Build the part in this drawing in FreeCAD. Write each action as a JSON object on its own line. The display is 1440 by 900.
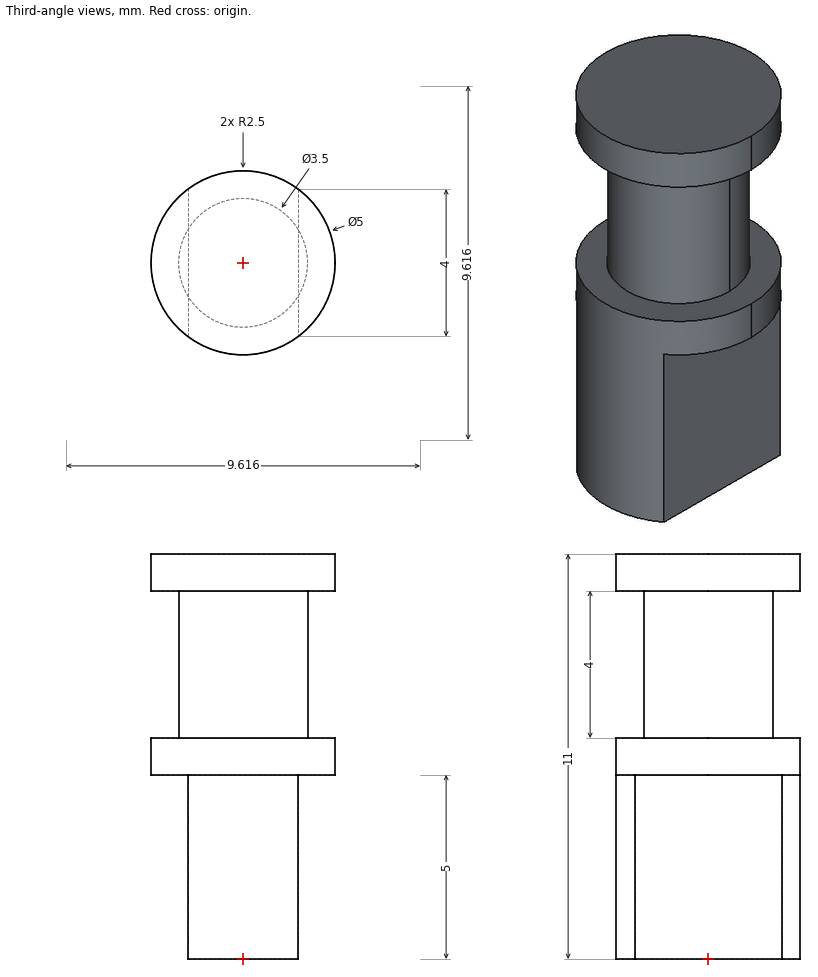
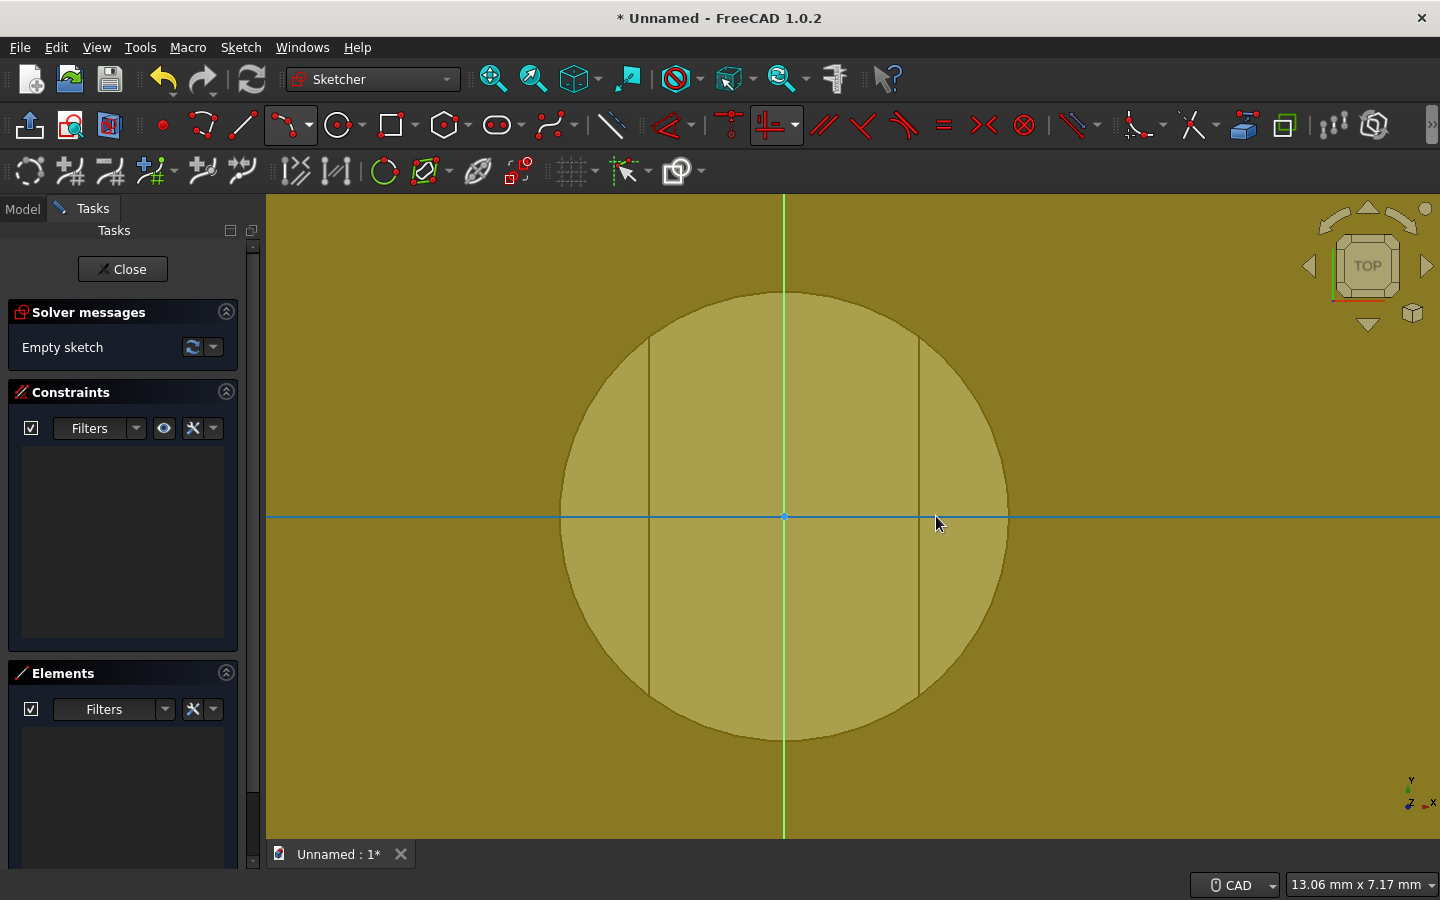
{"action": "key", "text": "g c"}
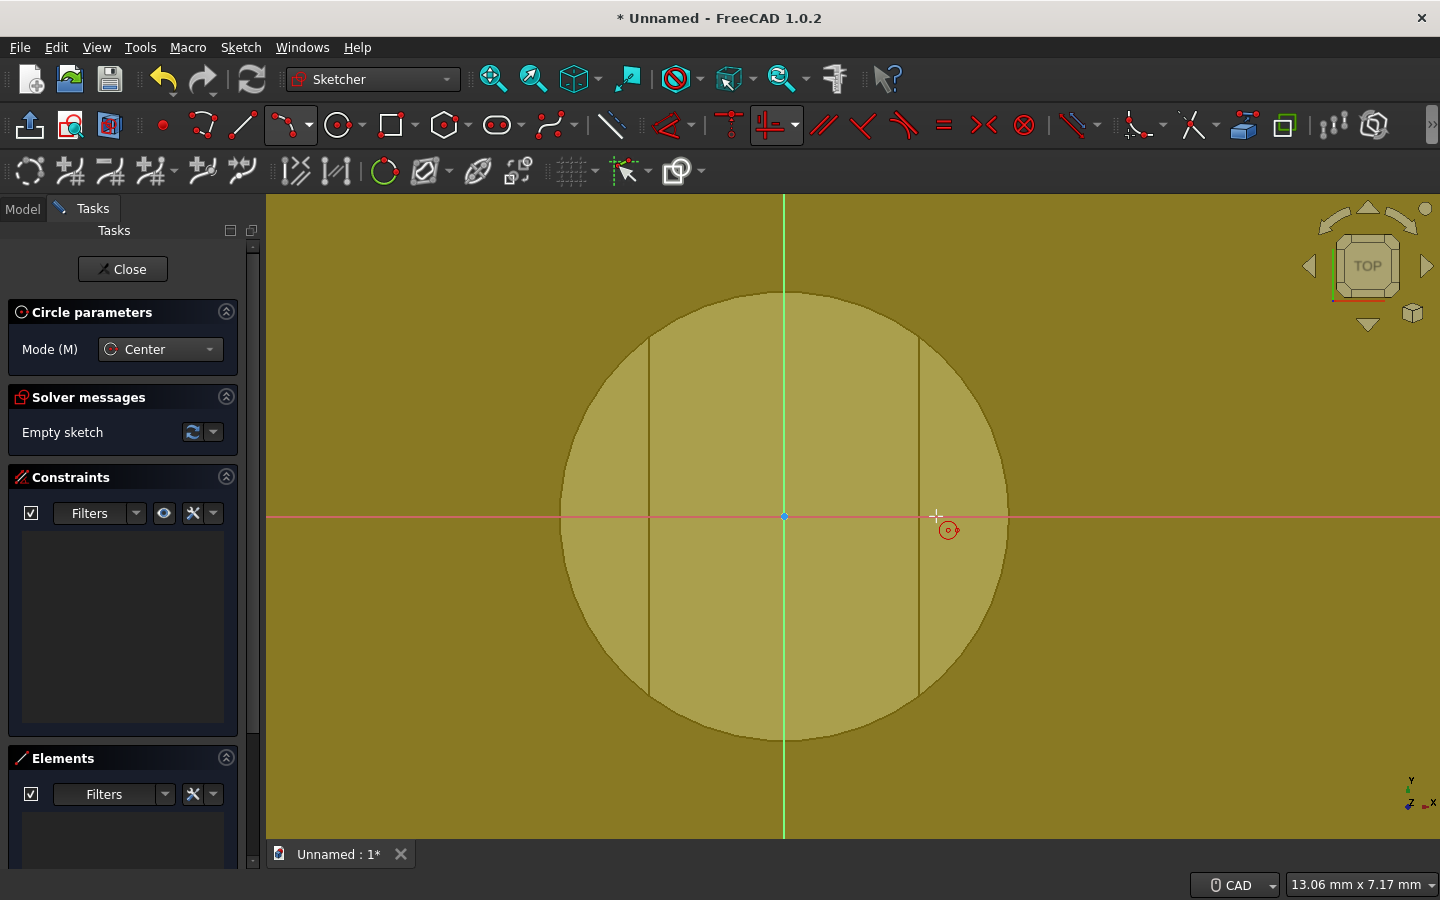
{"action": "left_click", "coordinate": [784, 516]}
{"action": "mouse_move", "coordinate": [943, 358]}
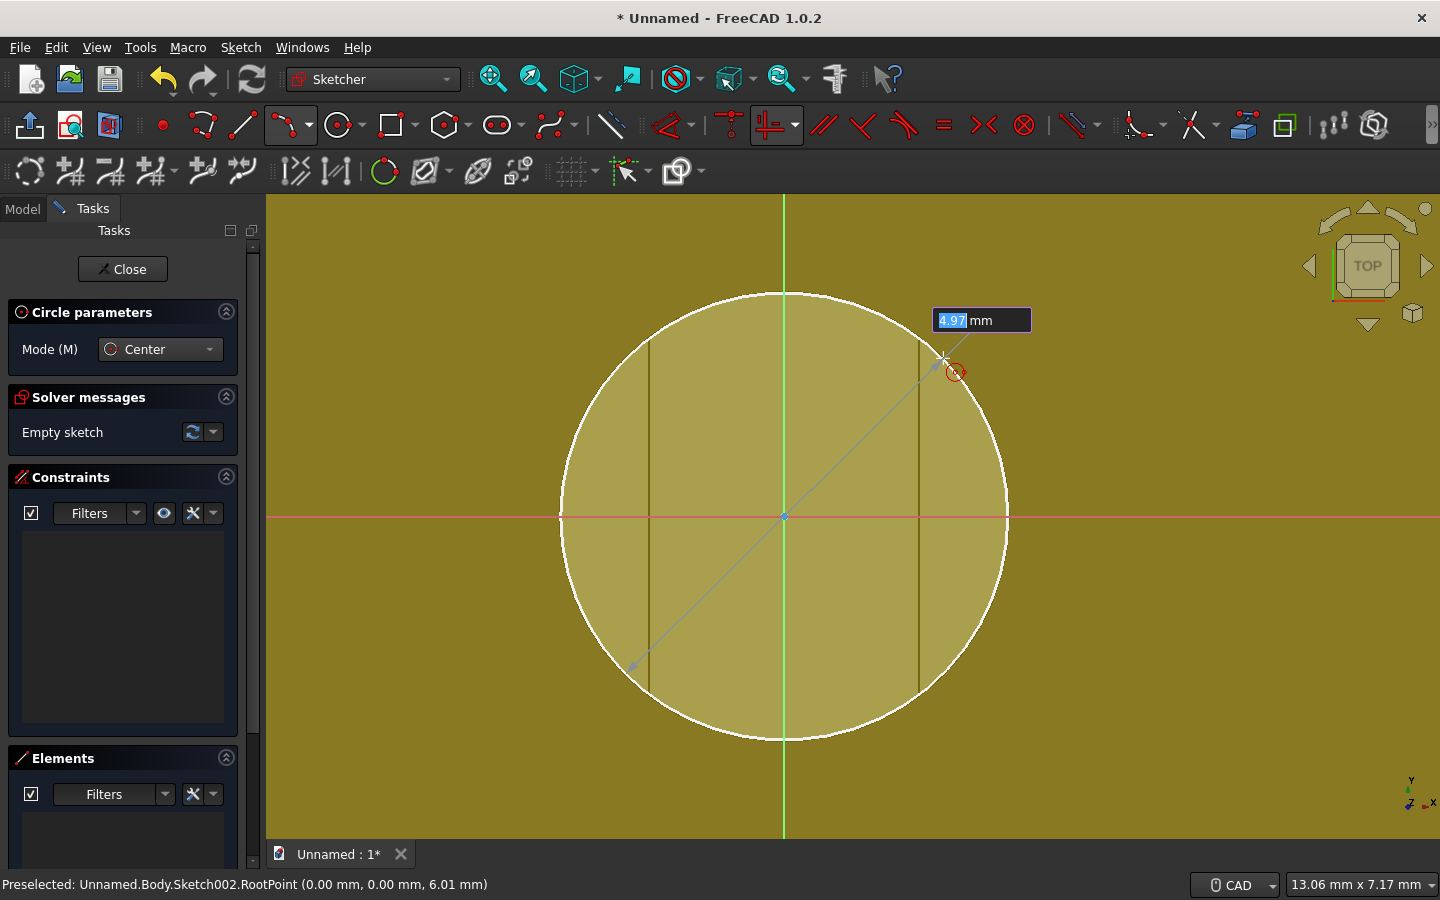
{"action": "type", "text": "5"}
{"action": "key", "text": "Return"}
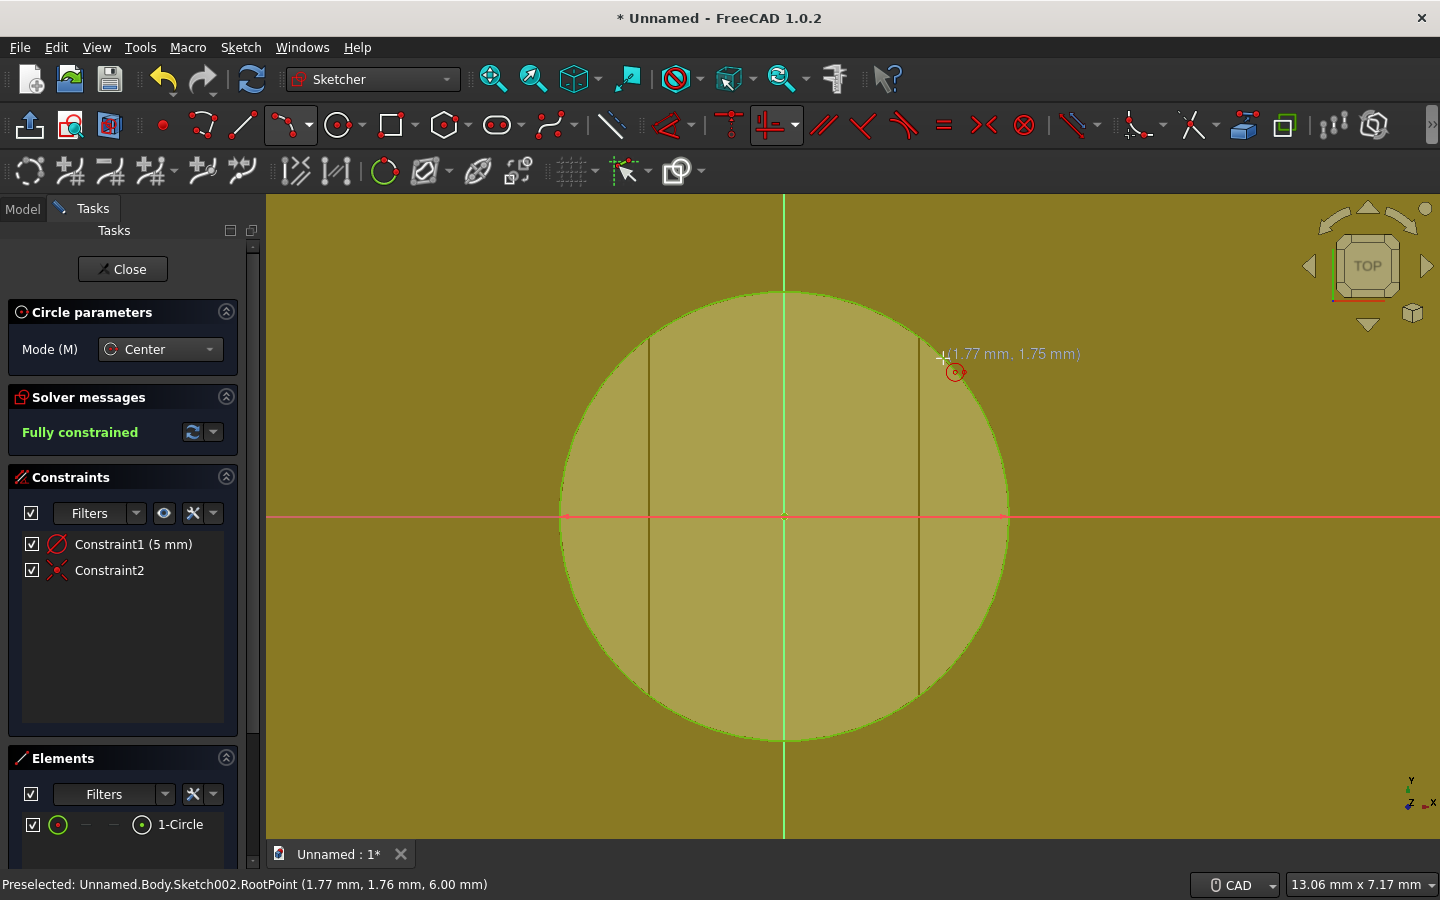
{"action": "left_click", "coordinate": [784, 516]}
{"action": "mouse_move", "coordinate": [896, 405]}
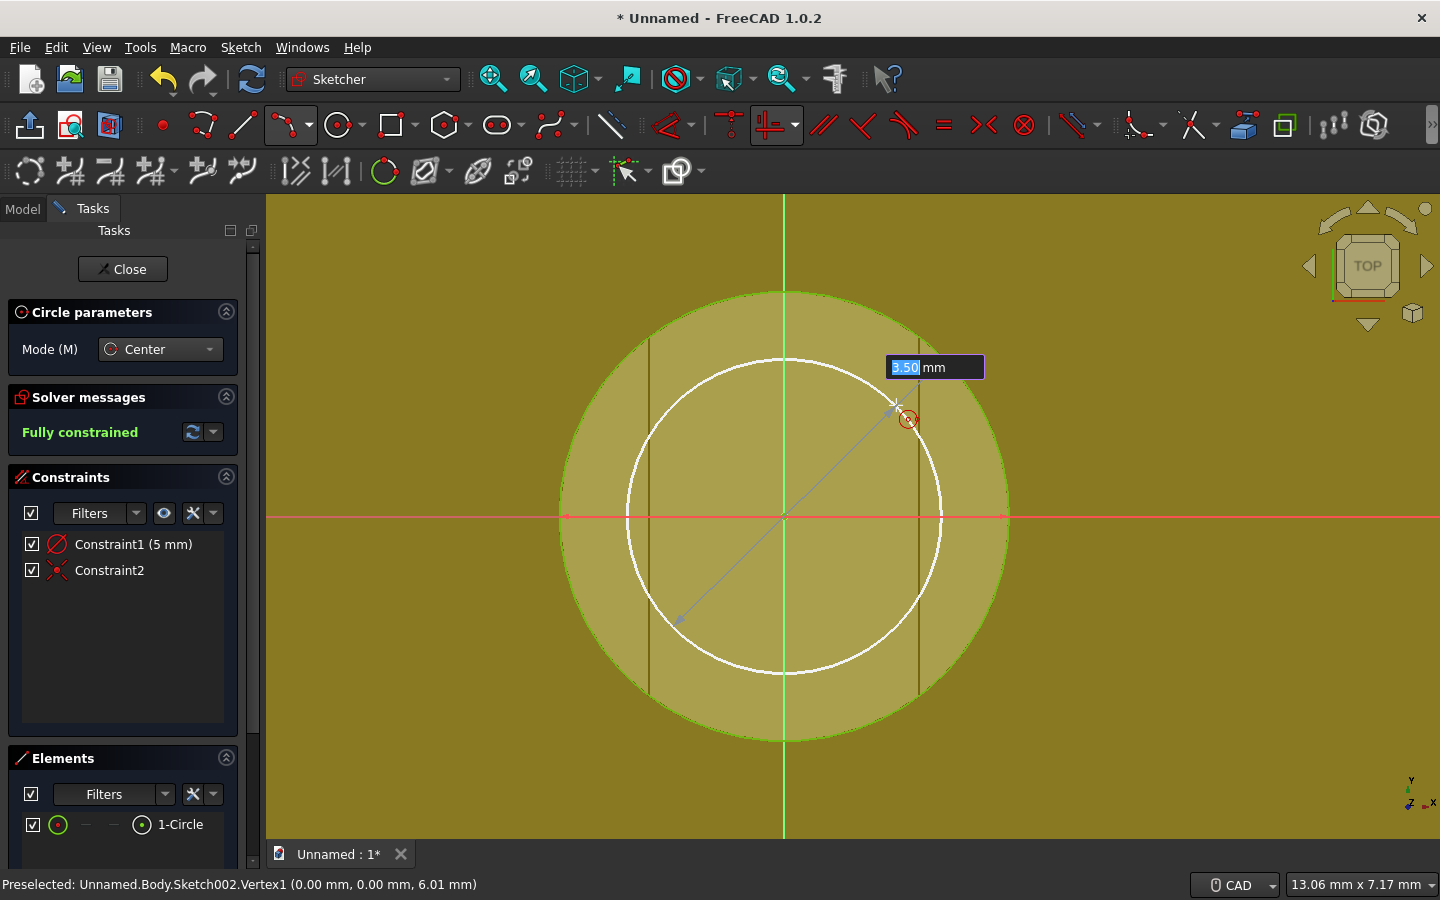
{"action": "type", "text": "3.5"}
{"action": "key", "text": "Return"}
{"action": "key", "text": "Escape"}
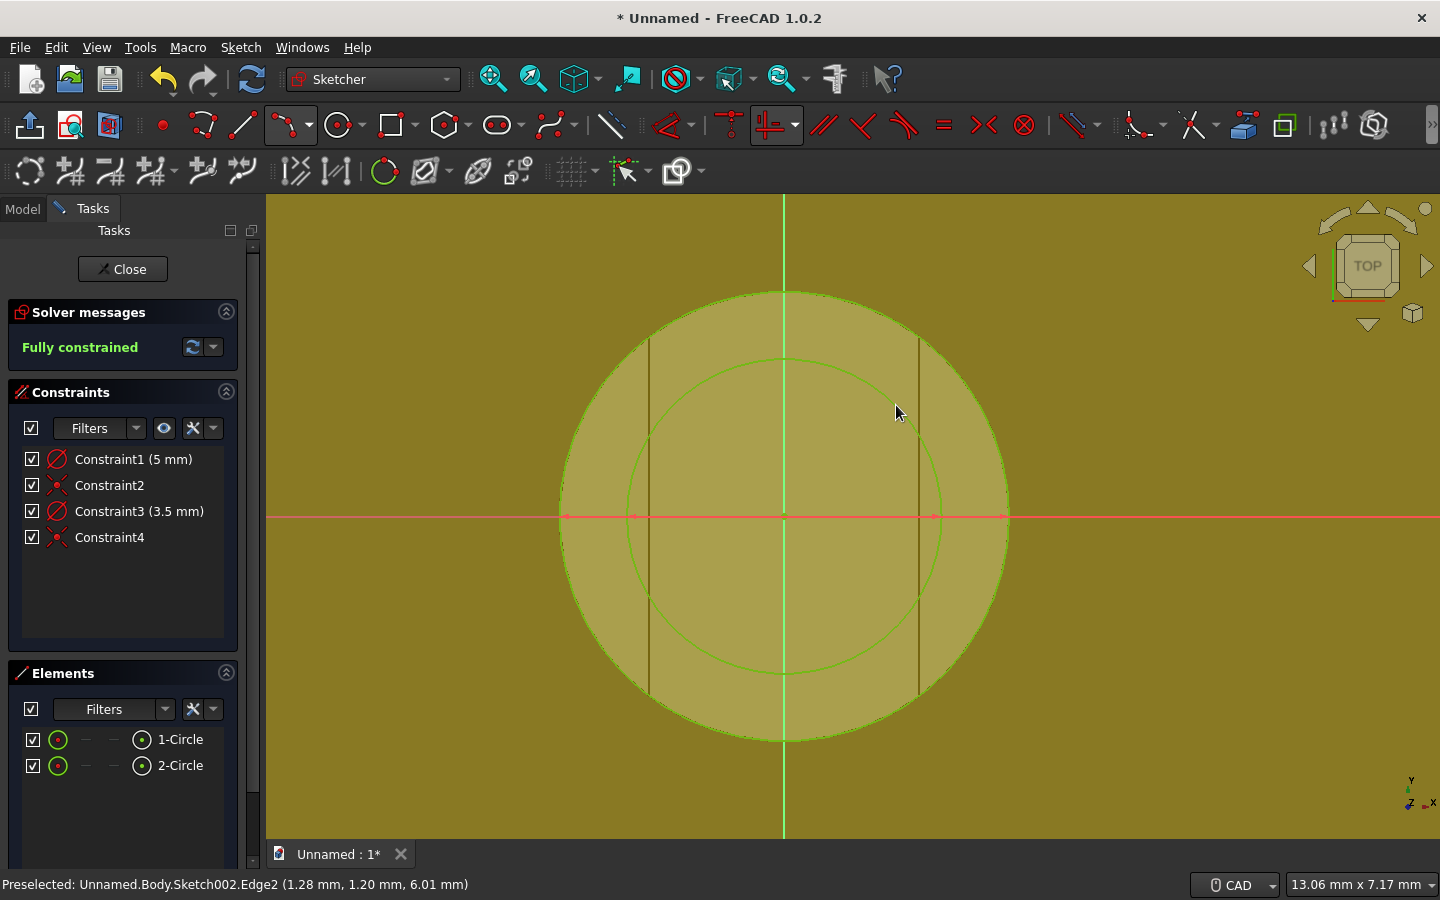
{"action": "left_click", "coordinate": [123, 269]}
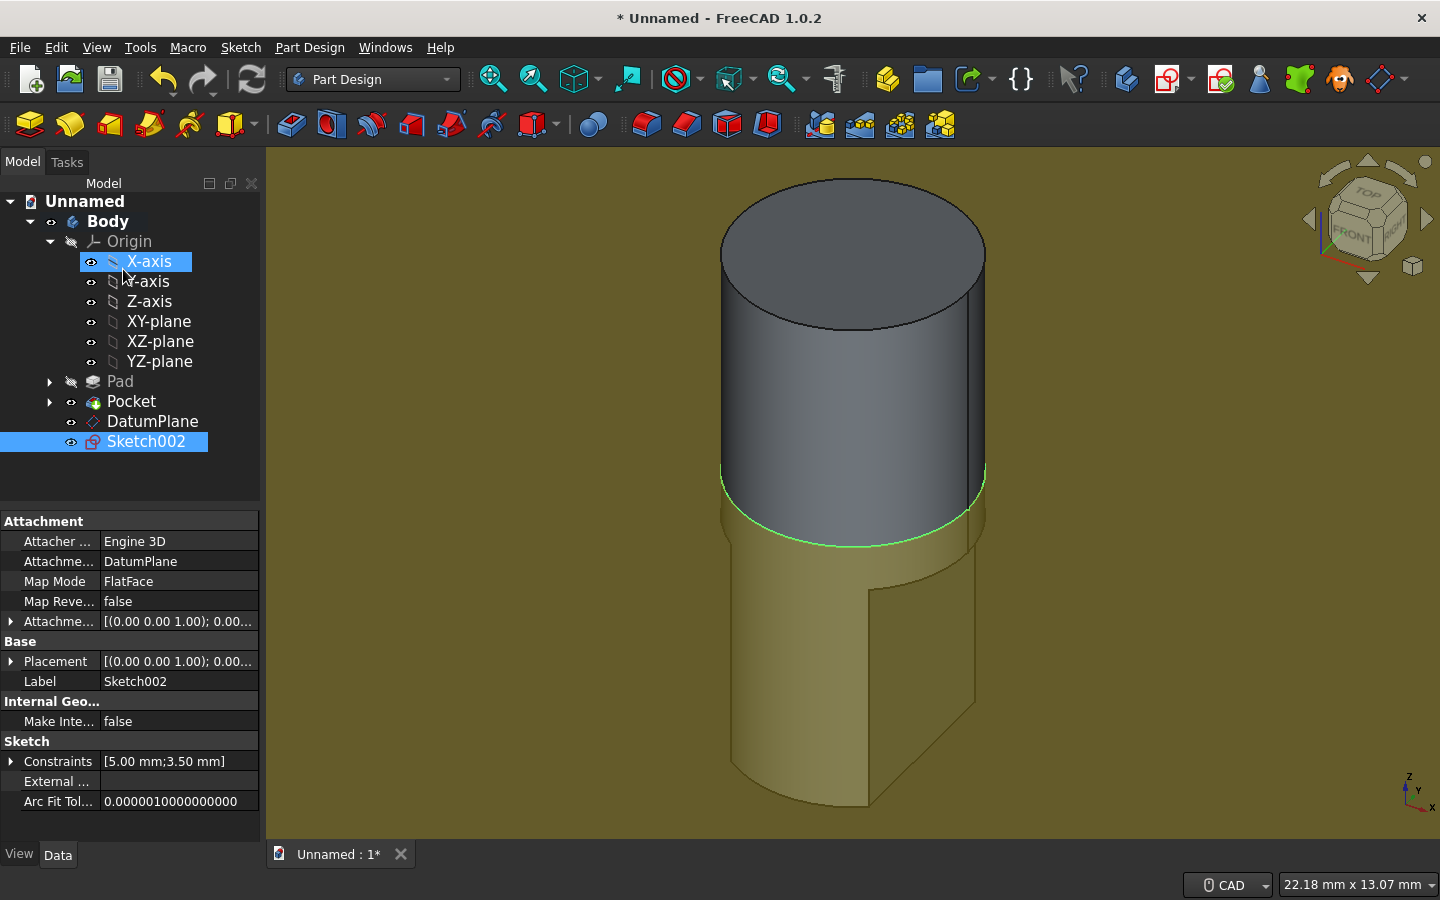
{"action": "left_click", "coordinate": [292, 124]}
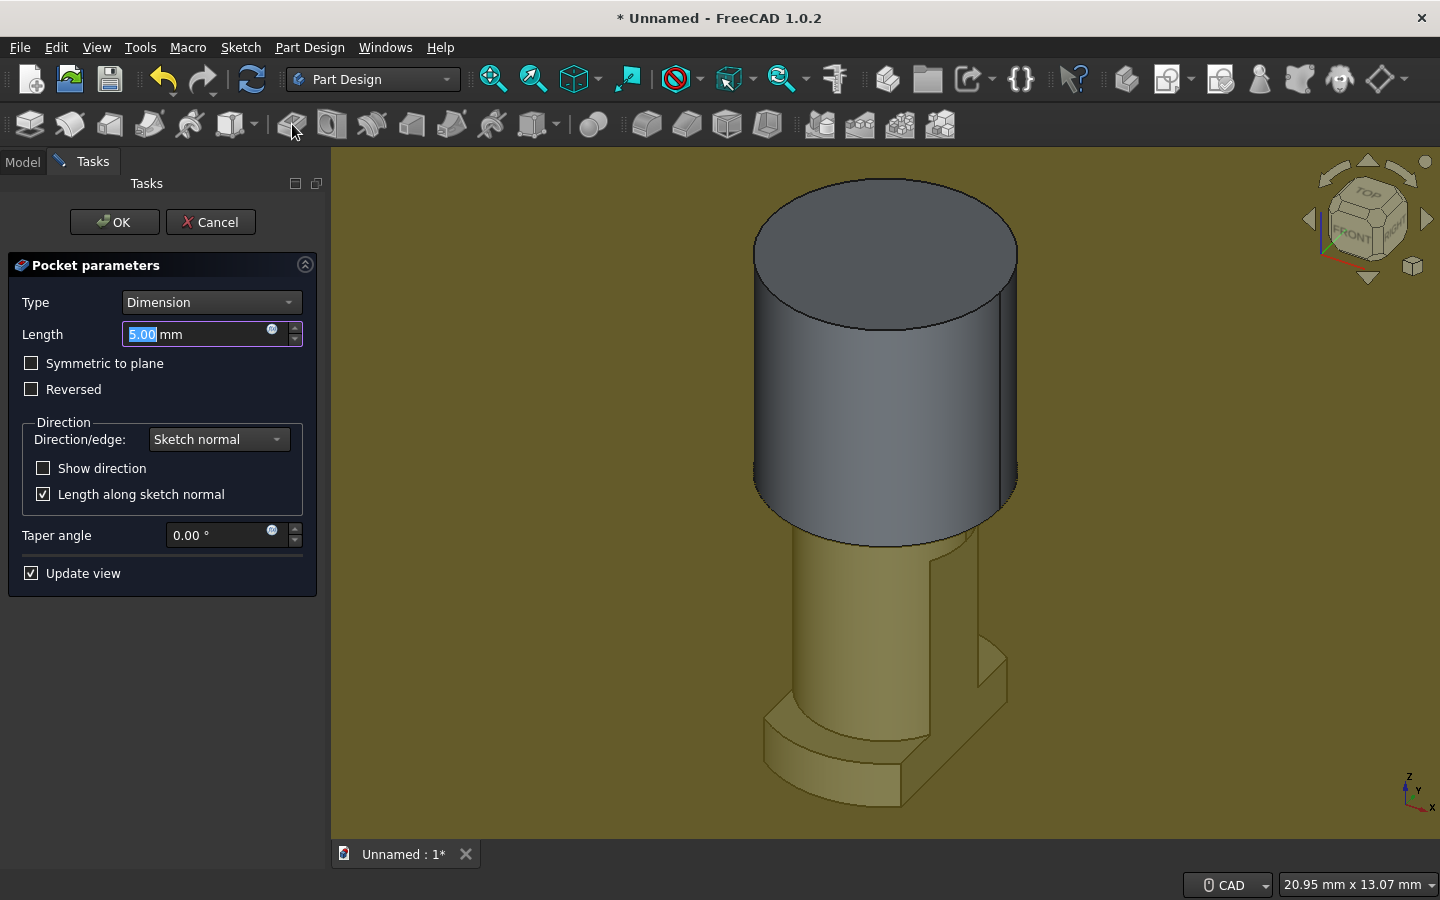
{"action": "type", "text": "4"}
{"action": "key", "text": "Tab"}